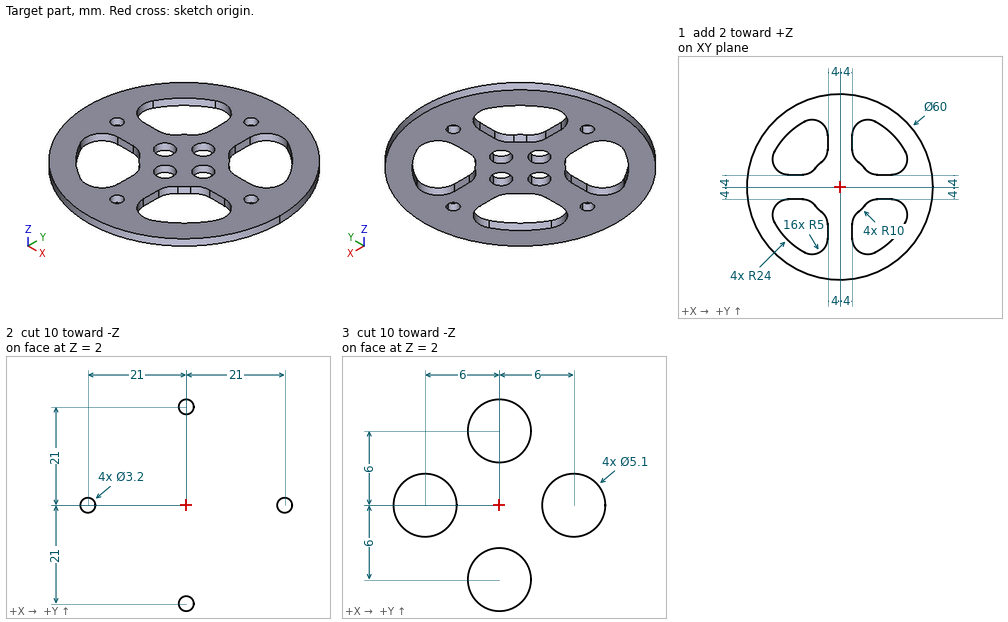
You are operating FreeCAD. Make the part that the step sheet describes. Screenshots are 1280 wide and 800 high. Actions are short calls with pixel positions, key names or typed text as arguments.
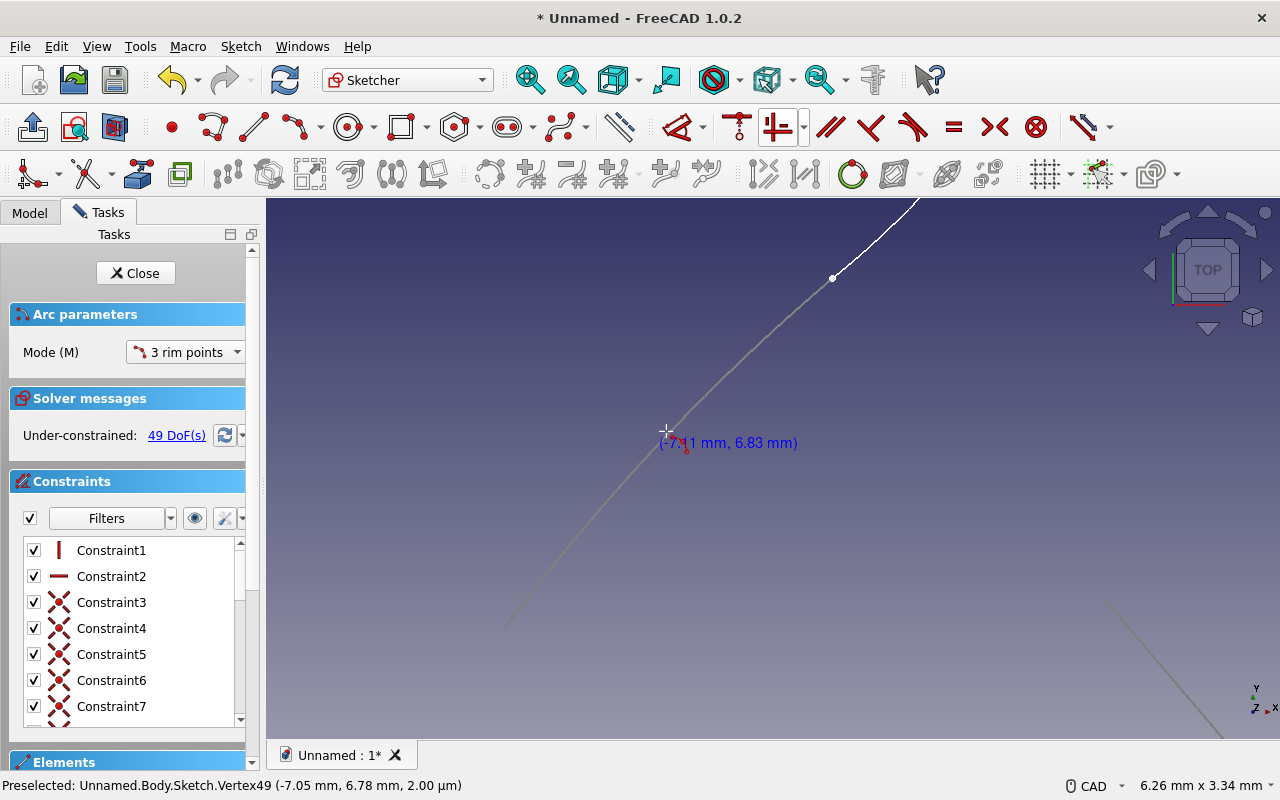
click(661, 410)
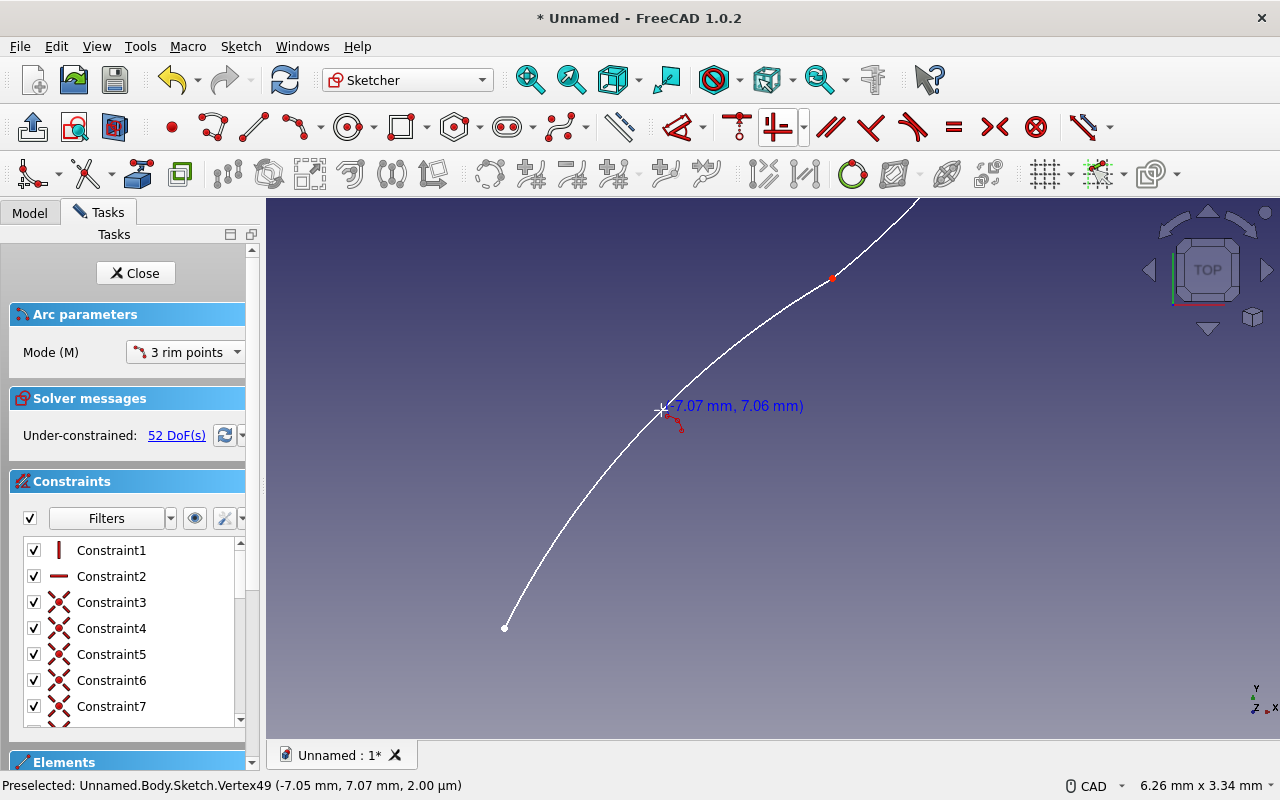
scroll(658, 422, down, 16)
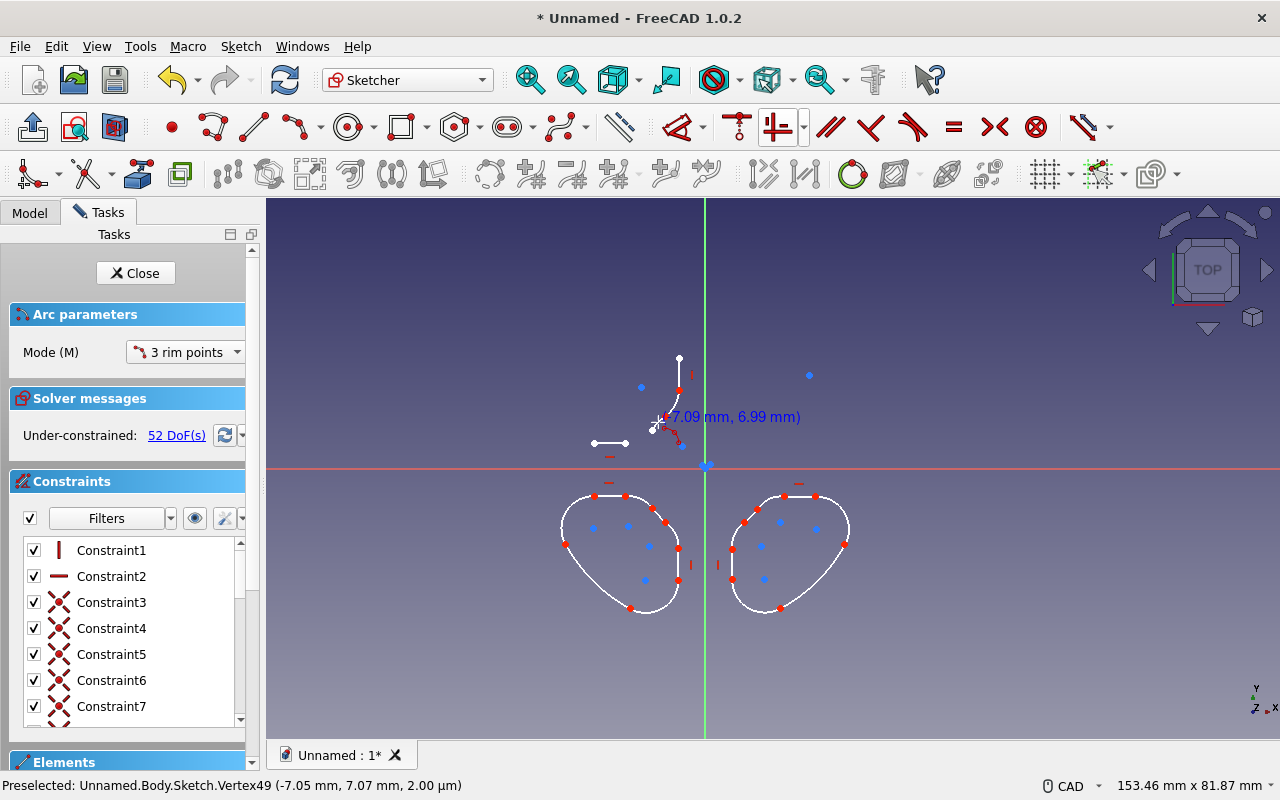
click(652, 431)
click(625, 443)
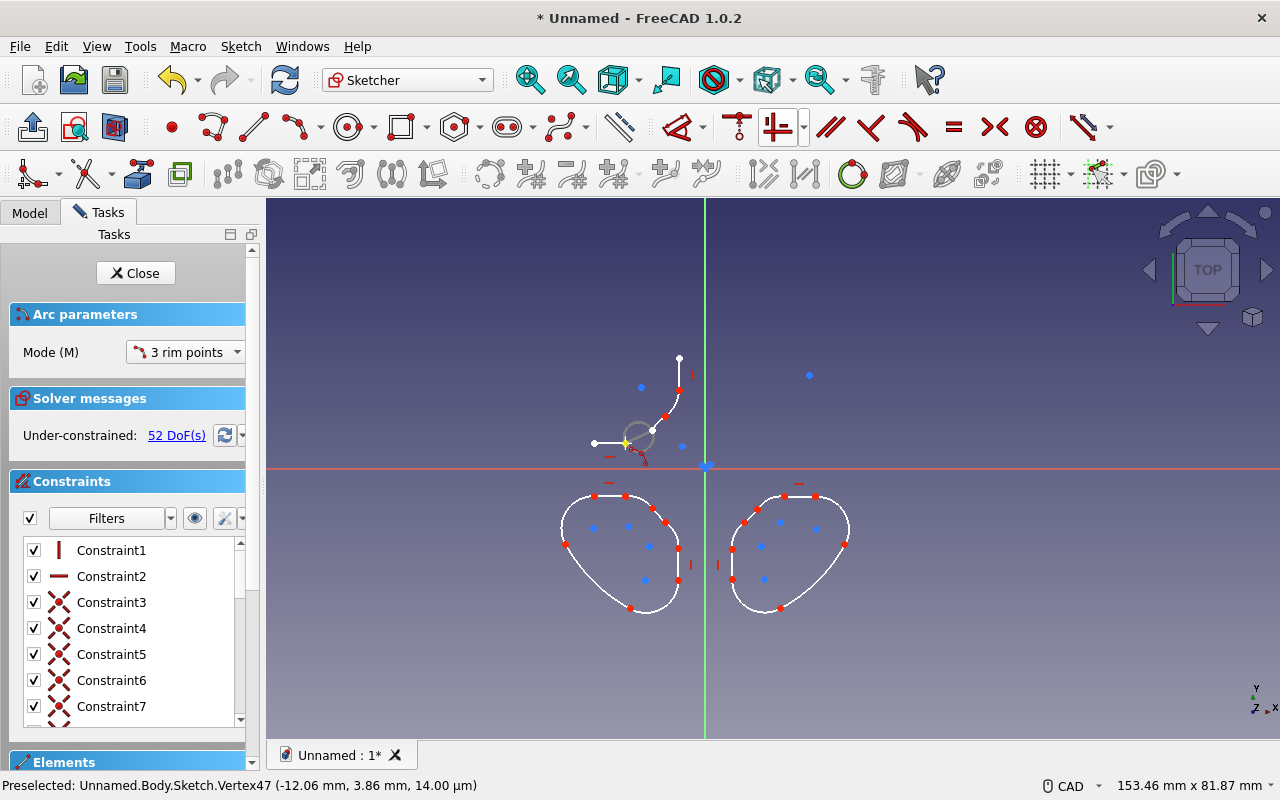
scroll(641, 439, up, 8)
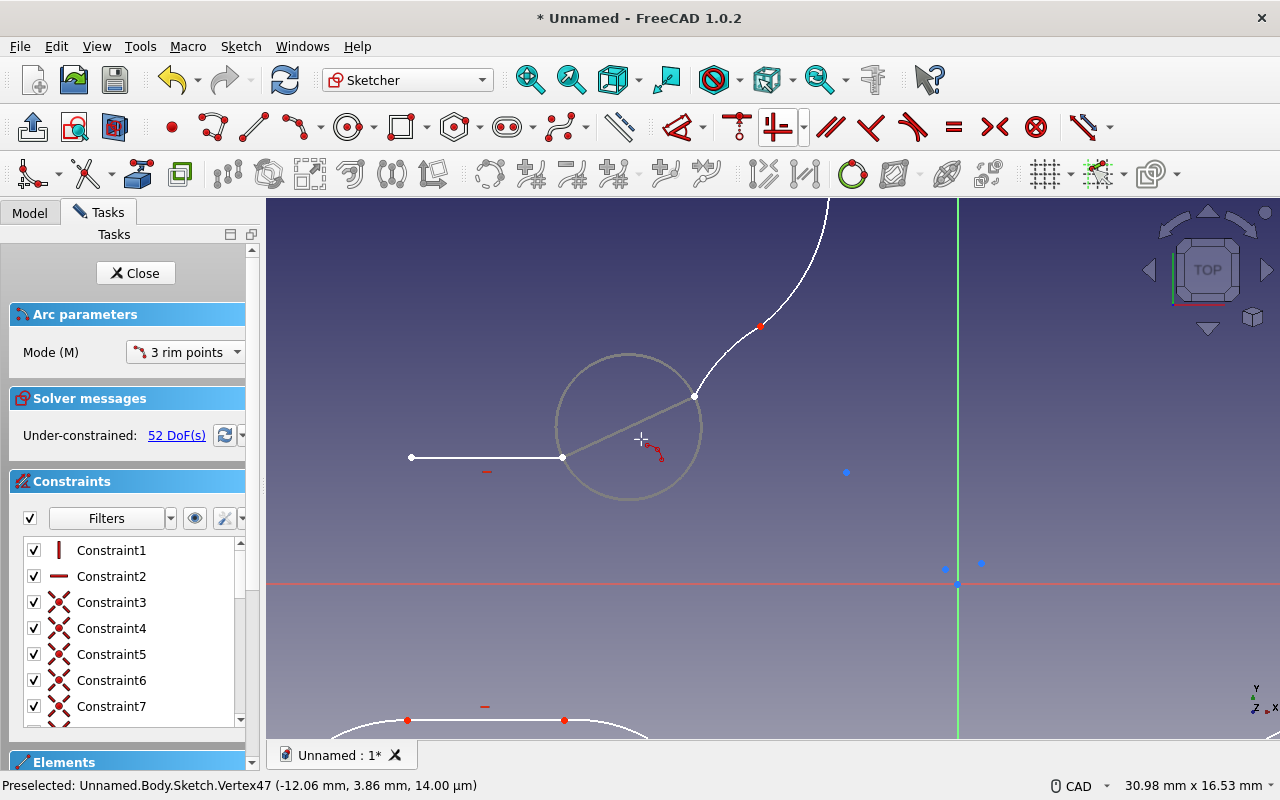
click(638, 436)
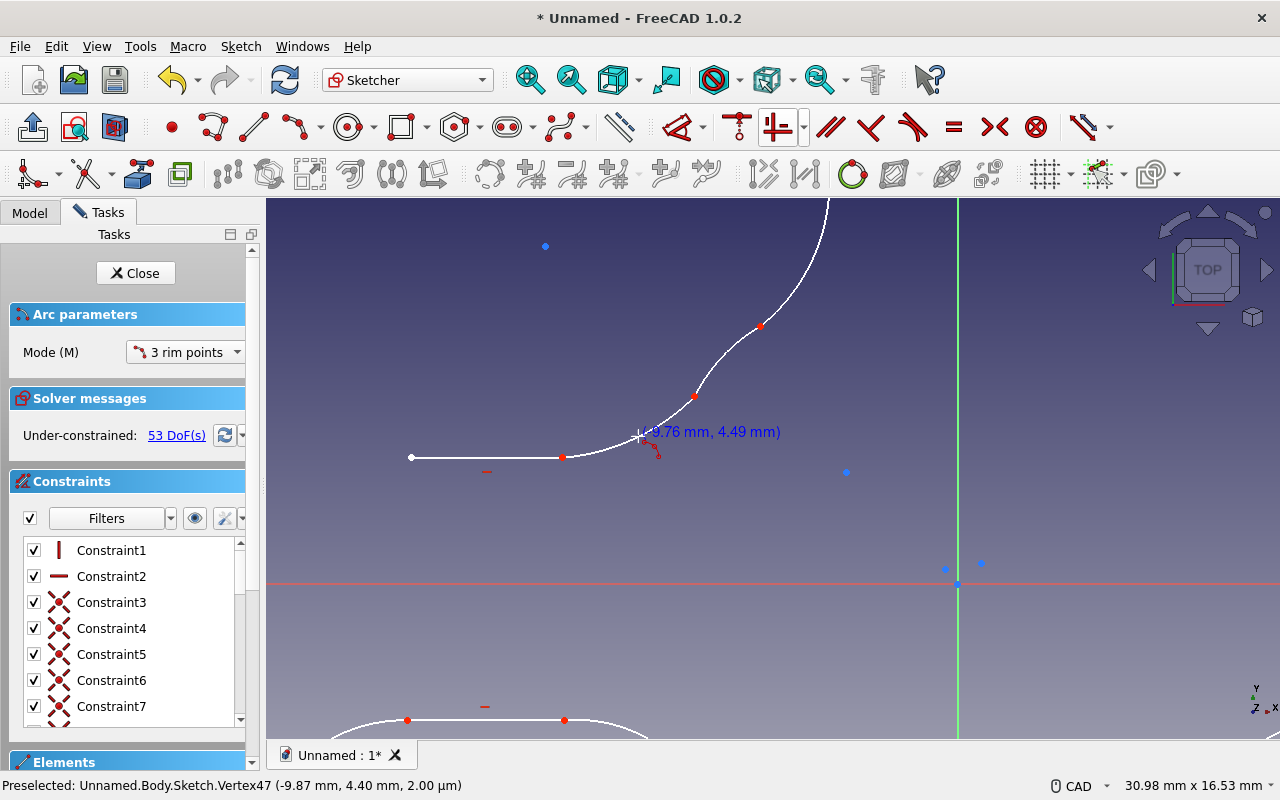
scroll(654, 446, down, 9)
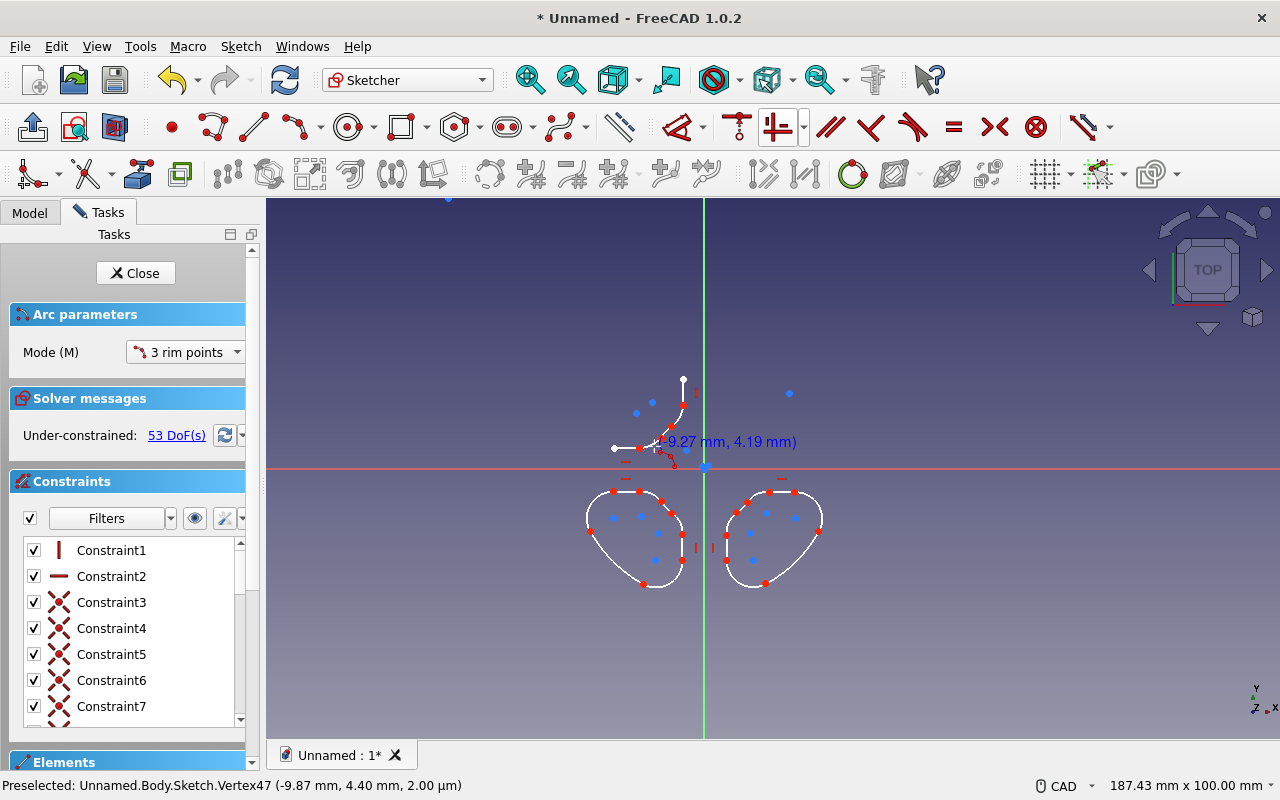
scroll(614, 448, up, 2)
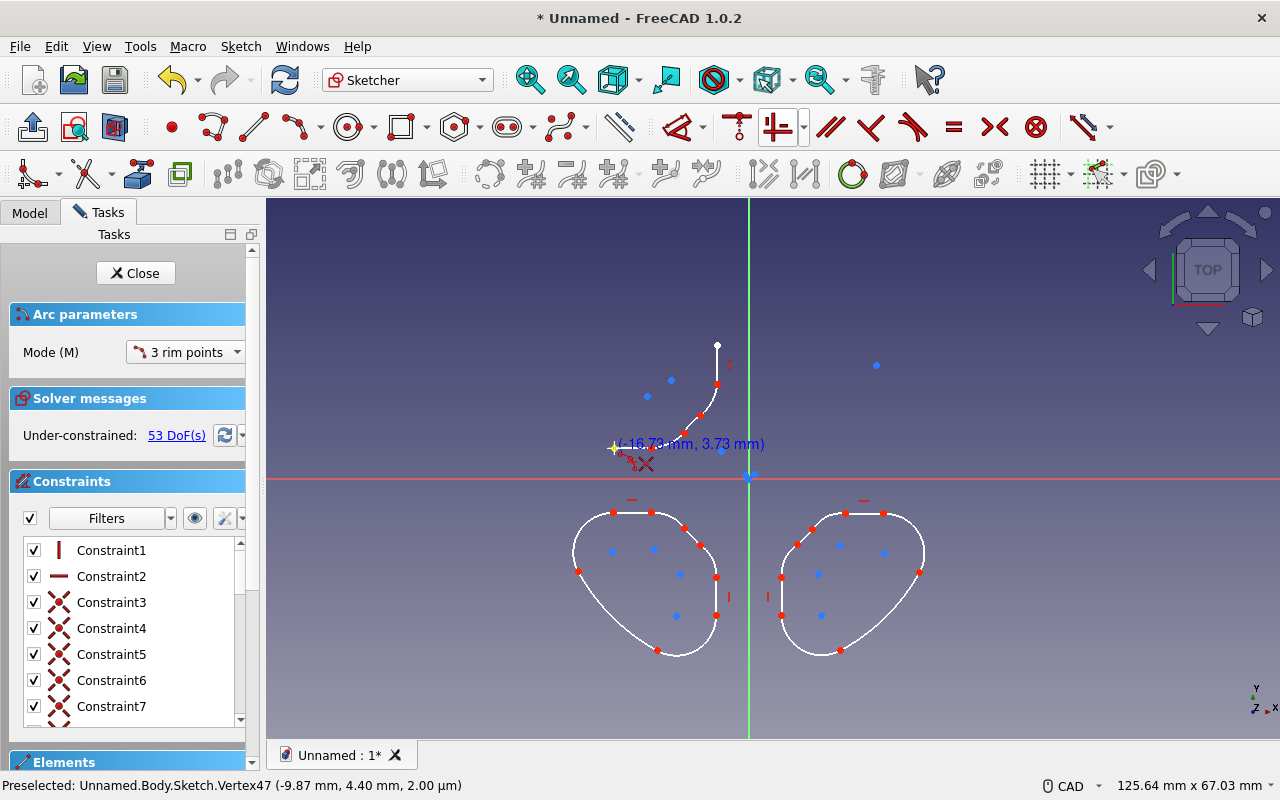
click(614, 448)
click(578, 388)
click(579, 427)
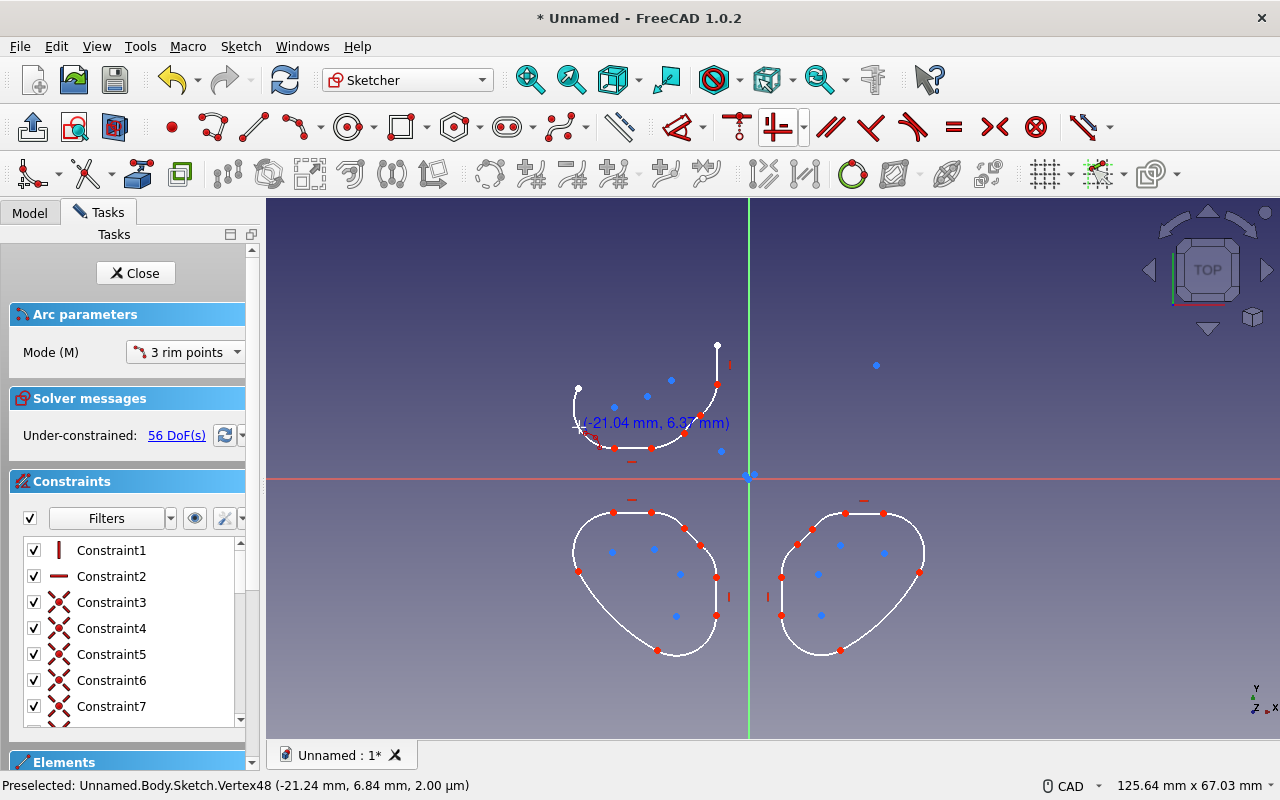
click(578, 389)
click(657, 309)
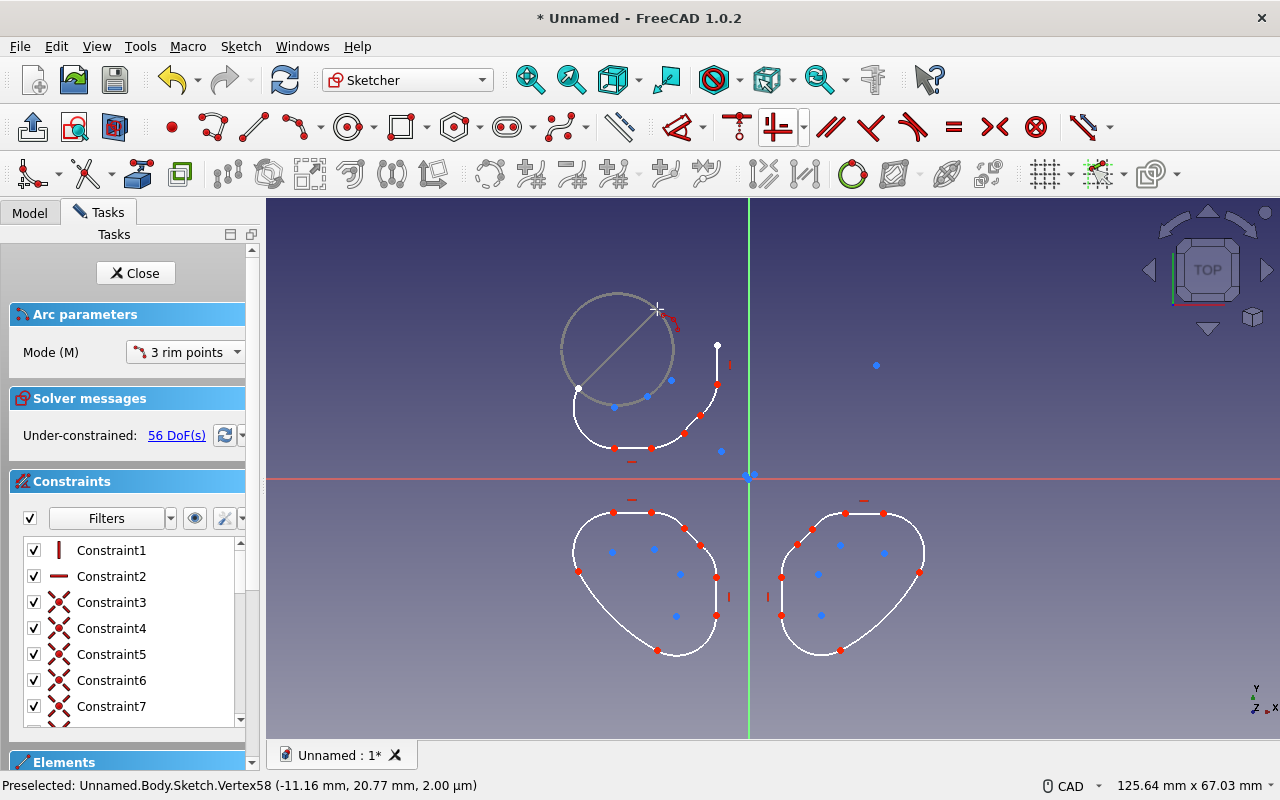
scroll(612, 342, up, 4)